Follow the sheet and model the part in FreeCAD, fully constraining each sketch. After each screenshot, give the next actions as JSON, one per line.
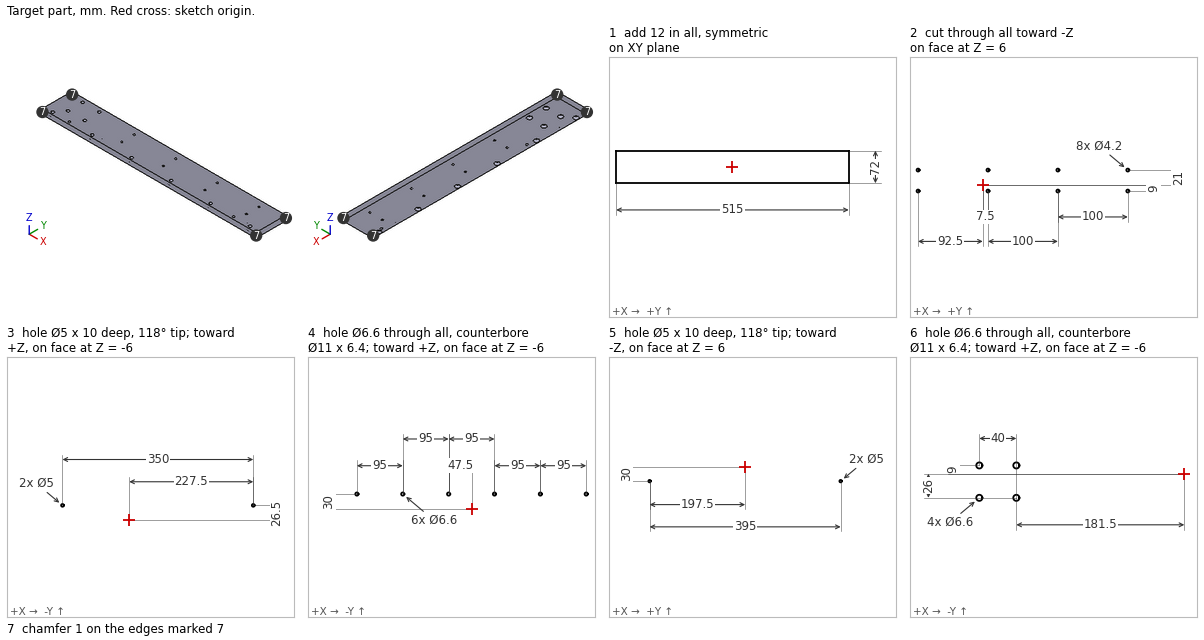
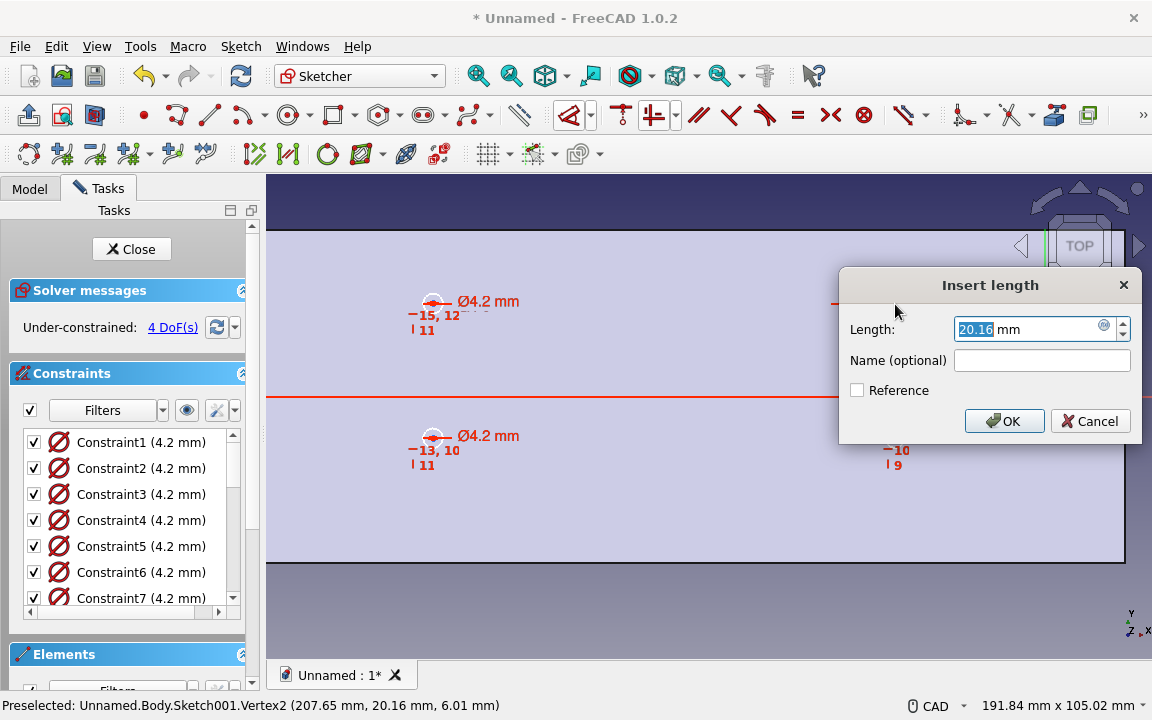
{"action": "type", "text": "21"}
{"action": "key", "text": "Return"}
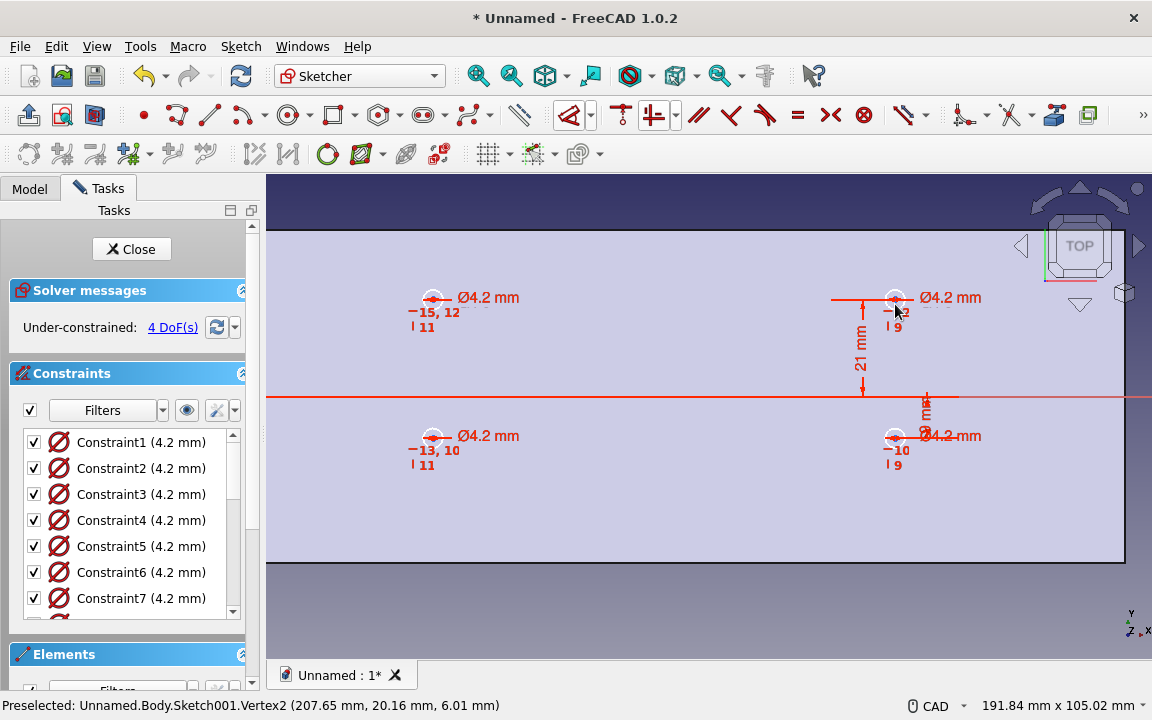
{"action": "scroll", "coordinate": [896, 444], "scroll_direction": "down", "scroll_amount": 5}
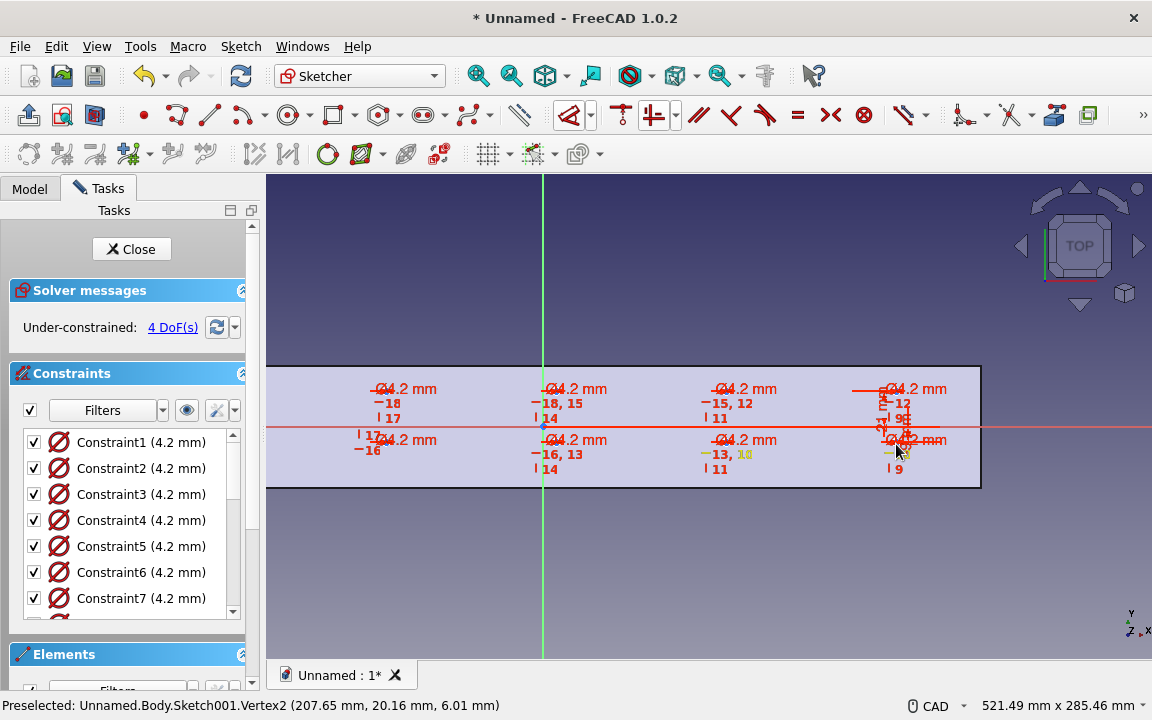
{"action": "scroll", "coordinate": [556, 442], "scroll_direction": "up", "scroll_amount": 6}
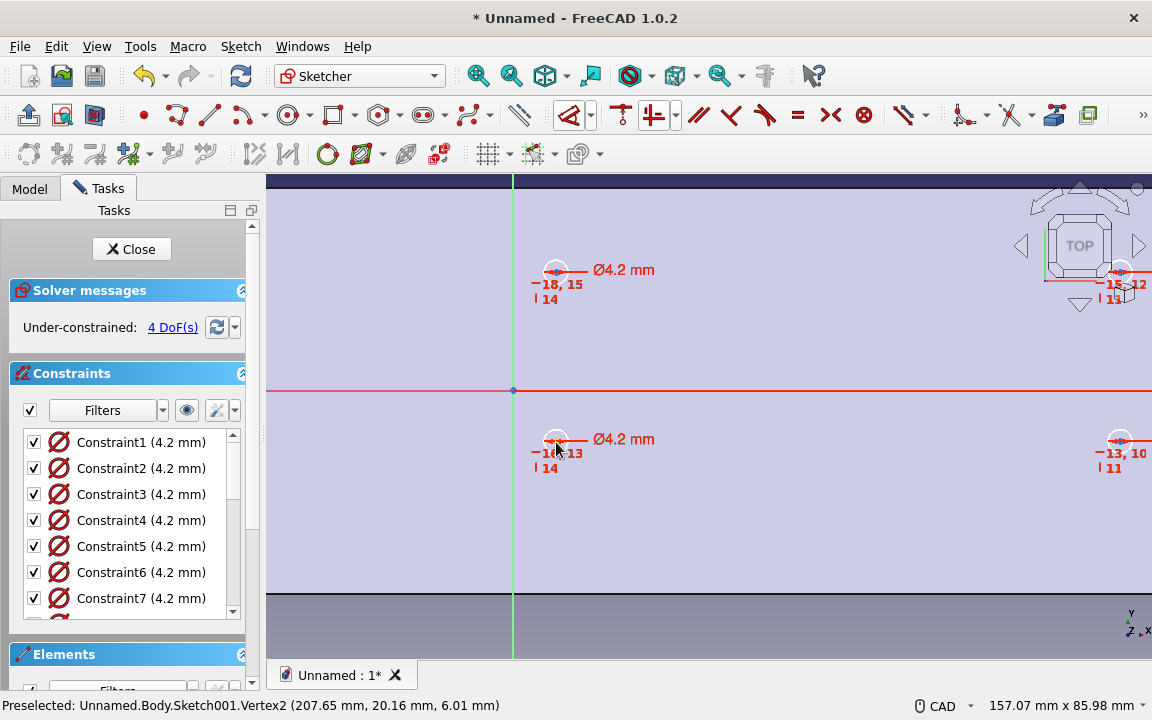
{"action": "left_click", "coordinate": [556, 441]}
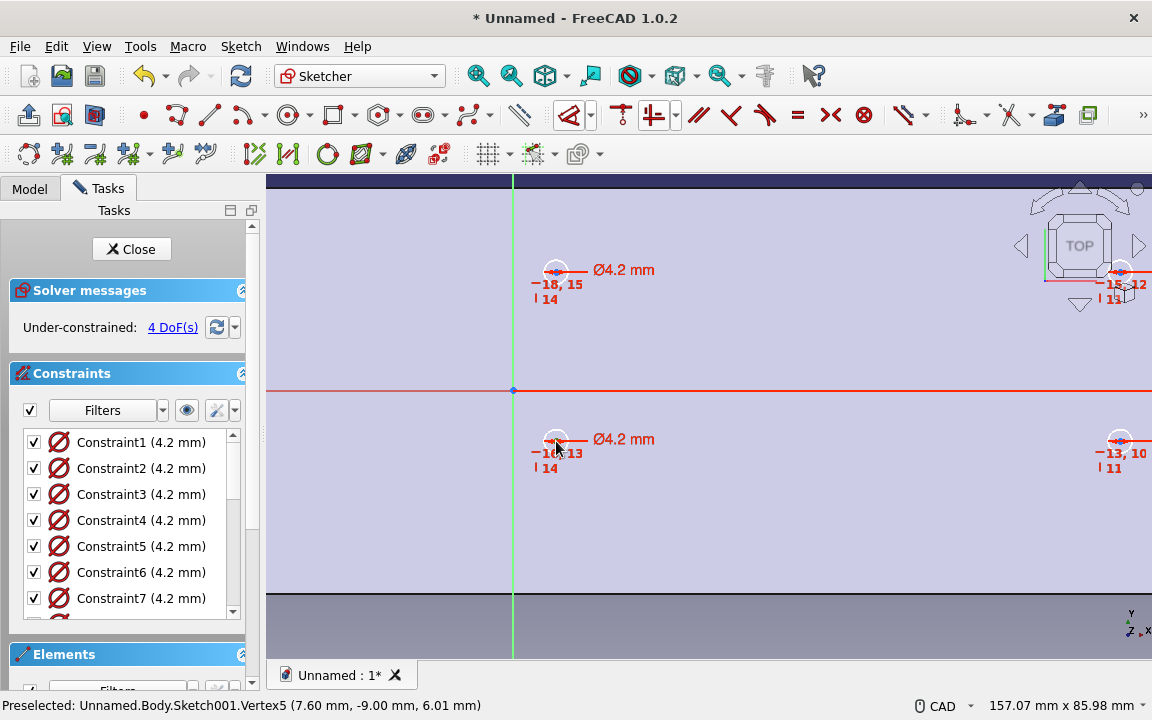
{"action": "key", "text": "l"}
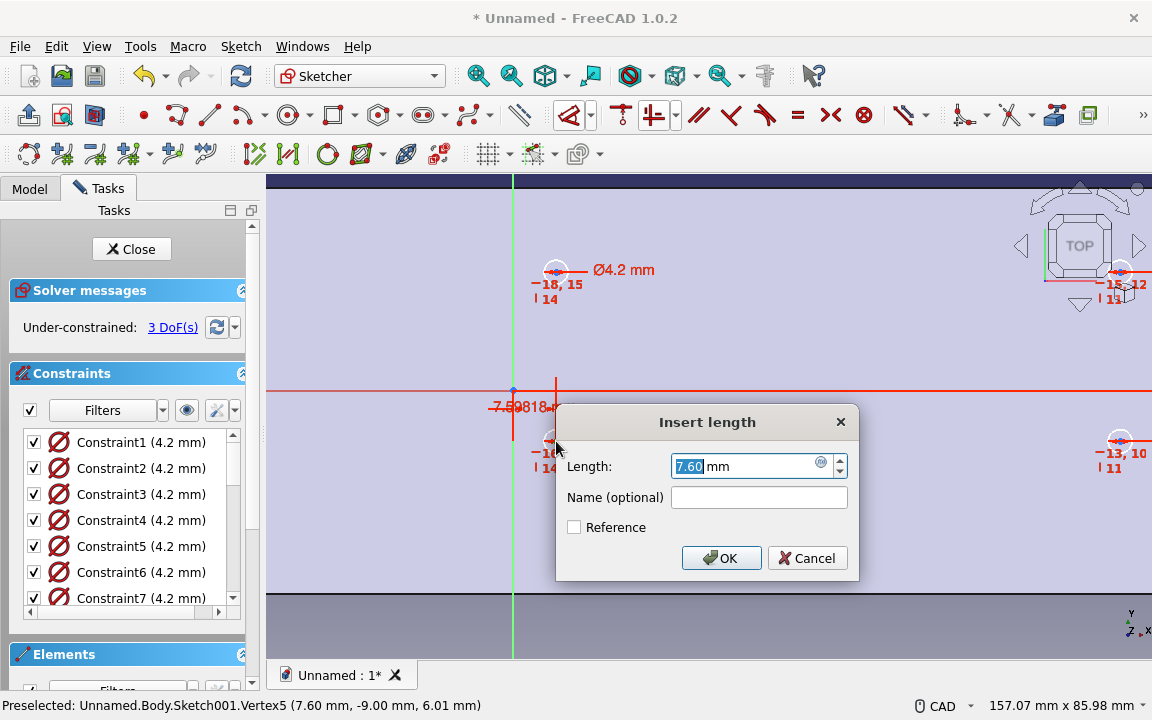
{"action": "type", "text": "7.5"}
{"action": "key", "text": "Return"}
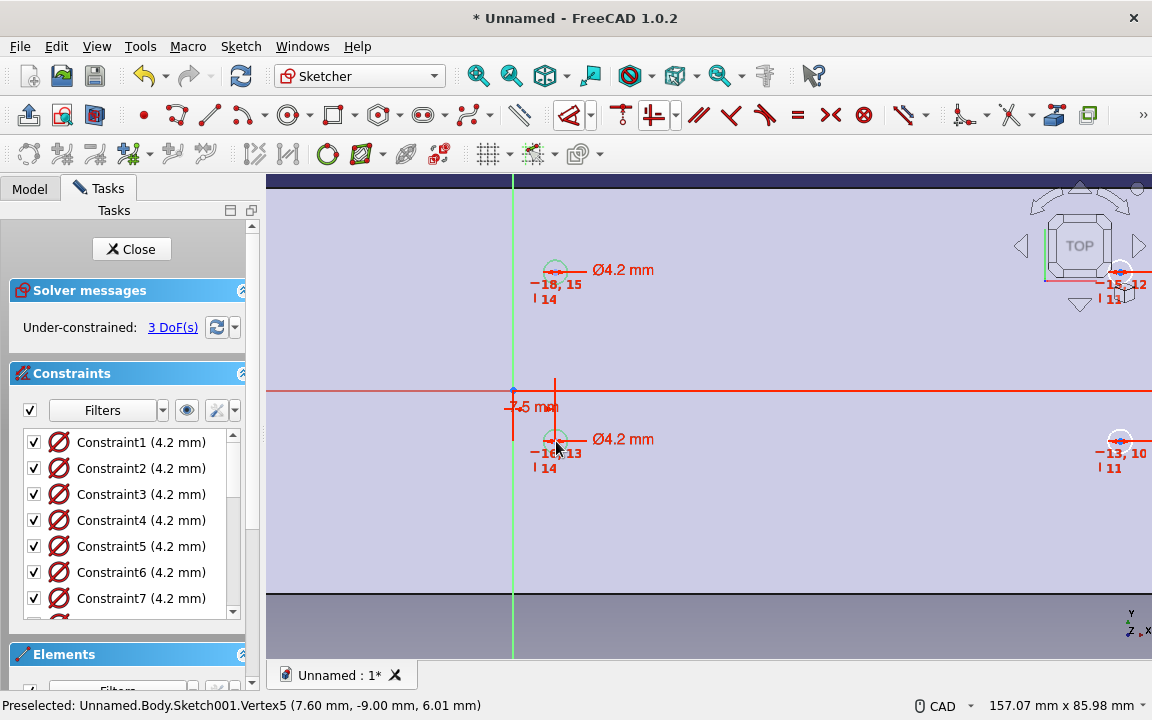
{"action": "scroll", "coordinate": [556, 442], "scroll_direction": "down", "scroll_amount": 6}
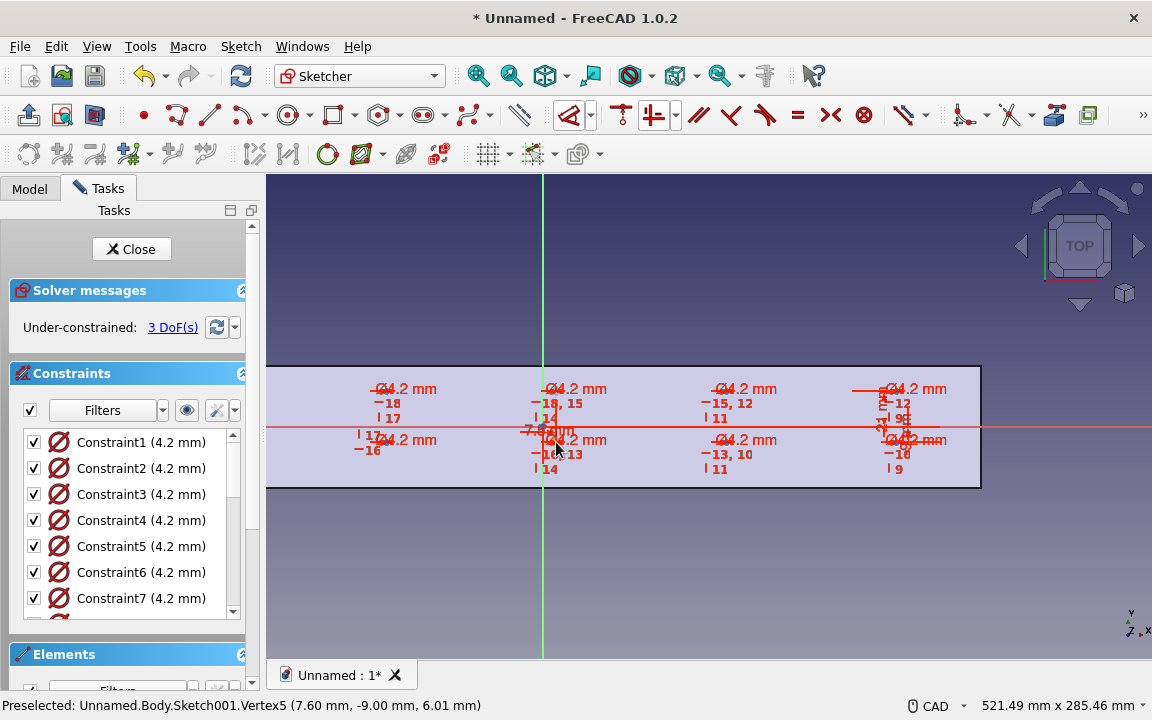
{"action": "left_click", "coordinate": [386, 442]}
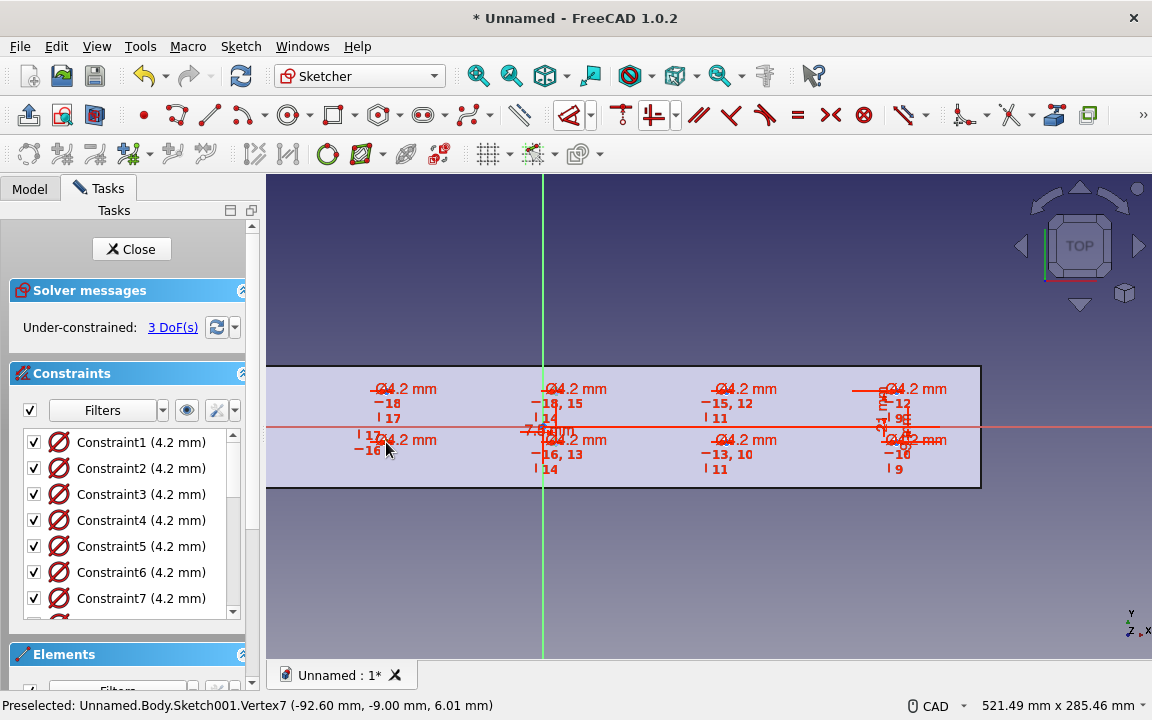
{"action": "left_click", "coordinate": [590, 116]}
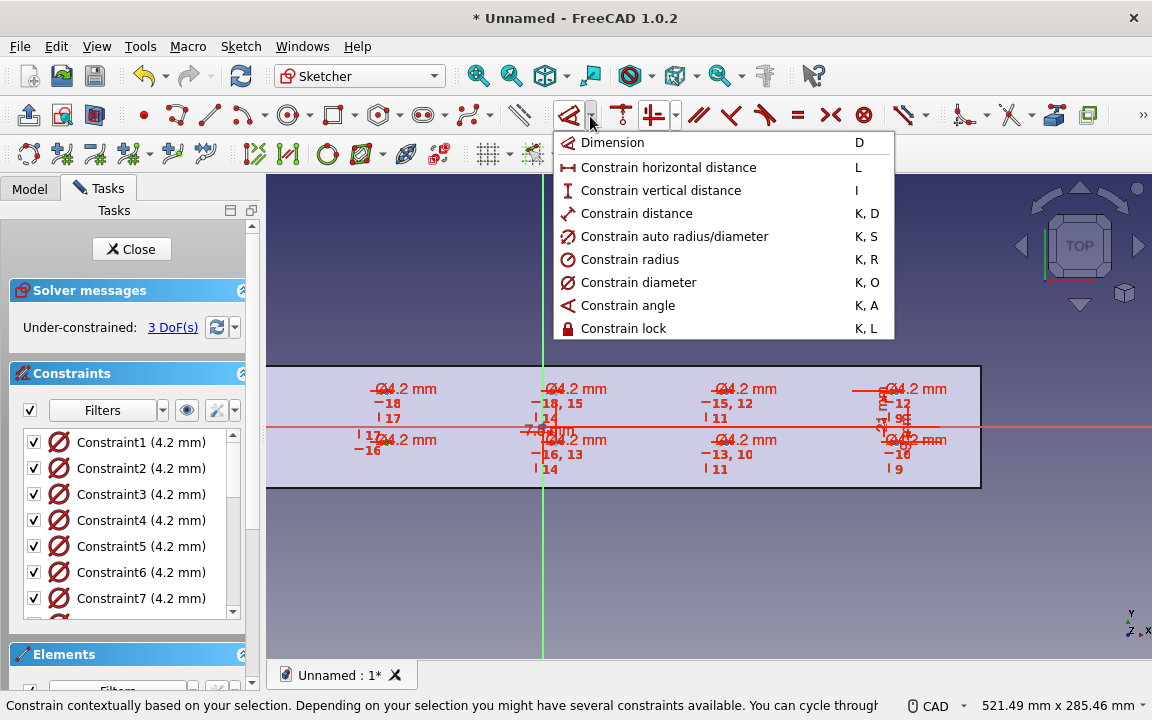
{"action": "left_click", "coordinate": [724, 168]}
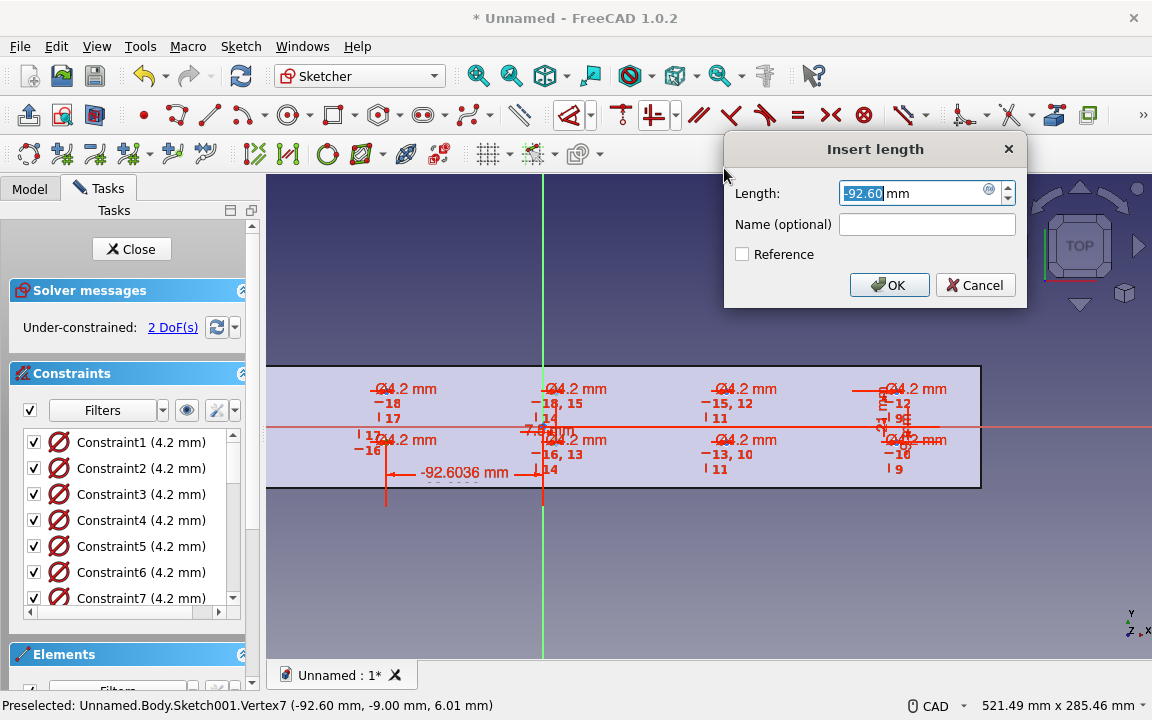
{"action": "type", "text": "-92.5"}
{"action": "key", "text": "Return"}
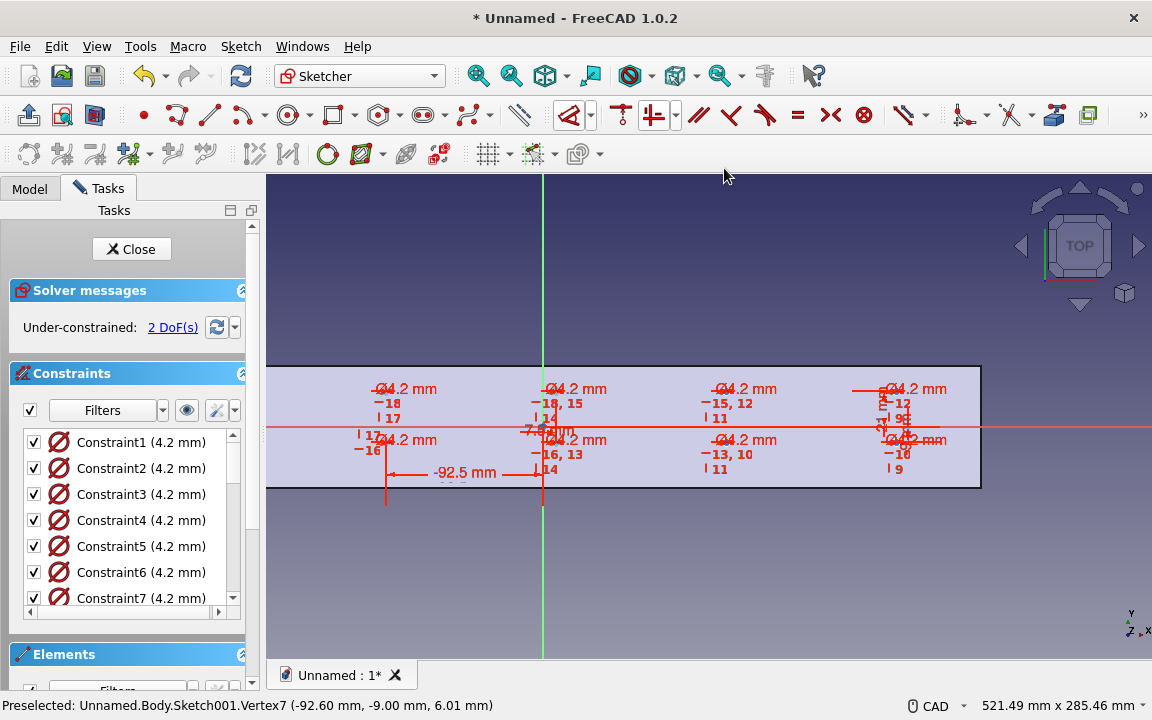
{"action": "left_click", "coordinate": [896, 442]}